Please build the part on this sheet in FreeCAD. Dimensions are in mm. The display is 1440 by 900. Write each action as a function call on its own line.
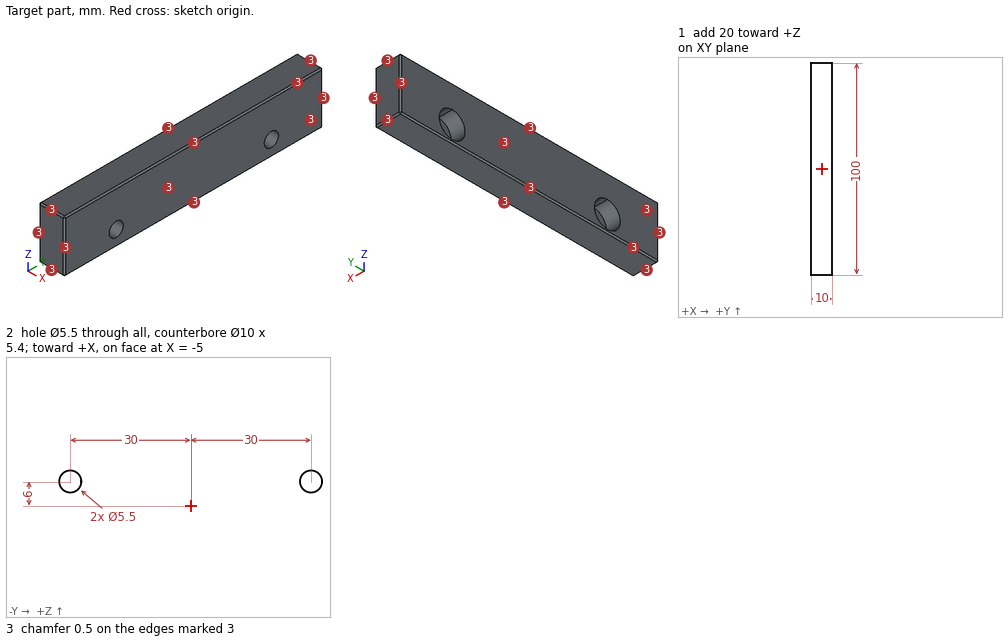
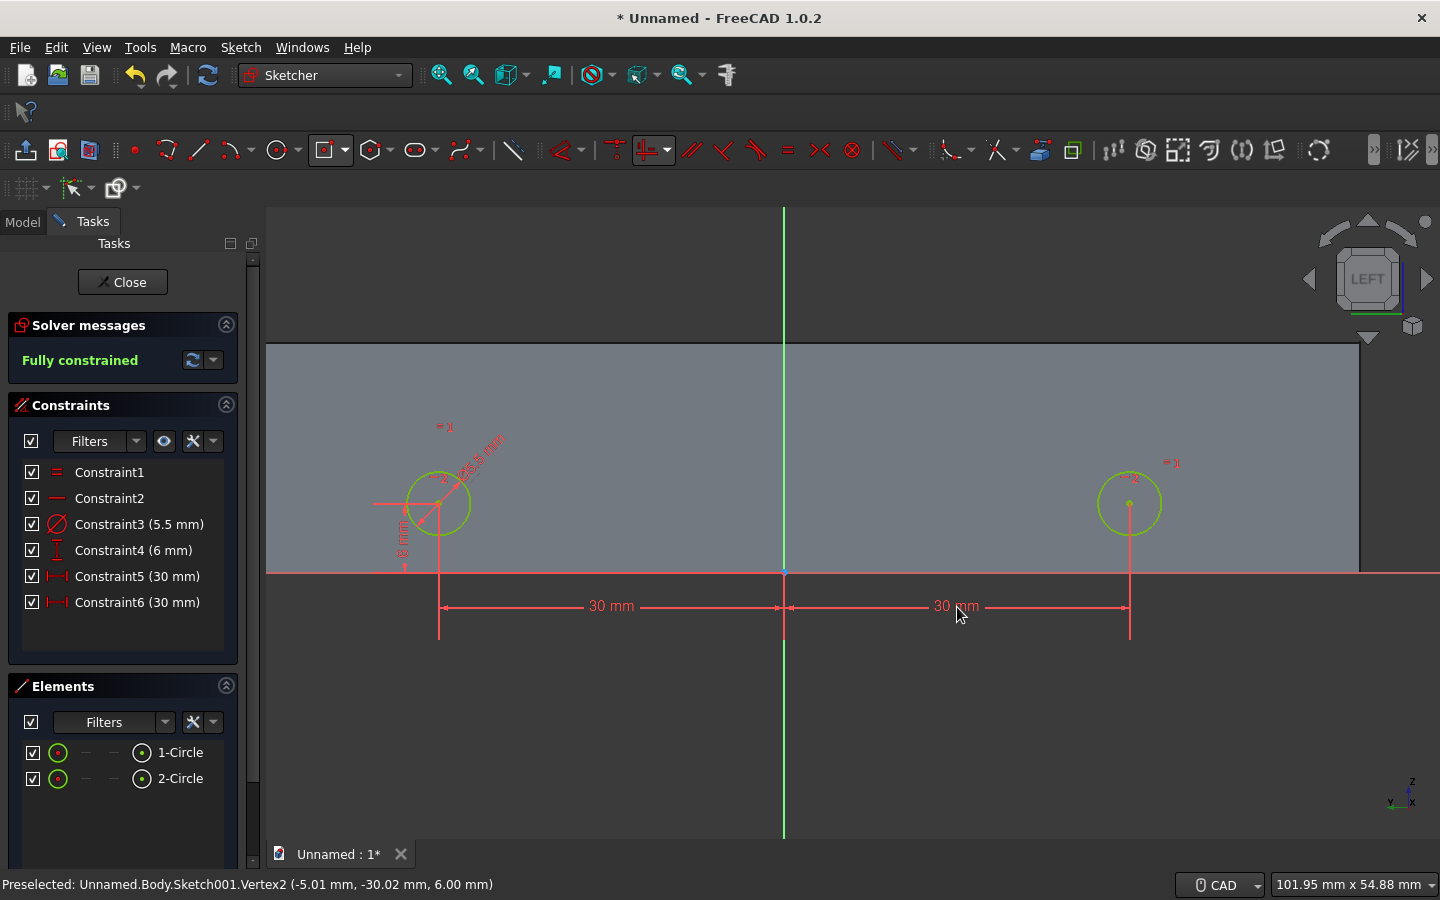
click(123, 282)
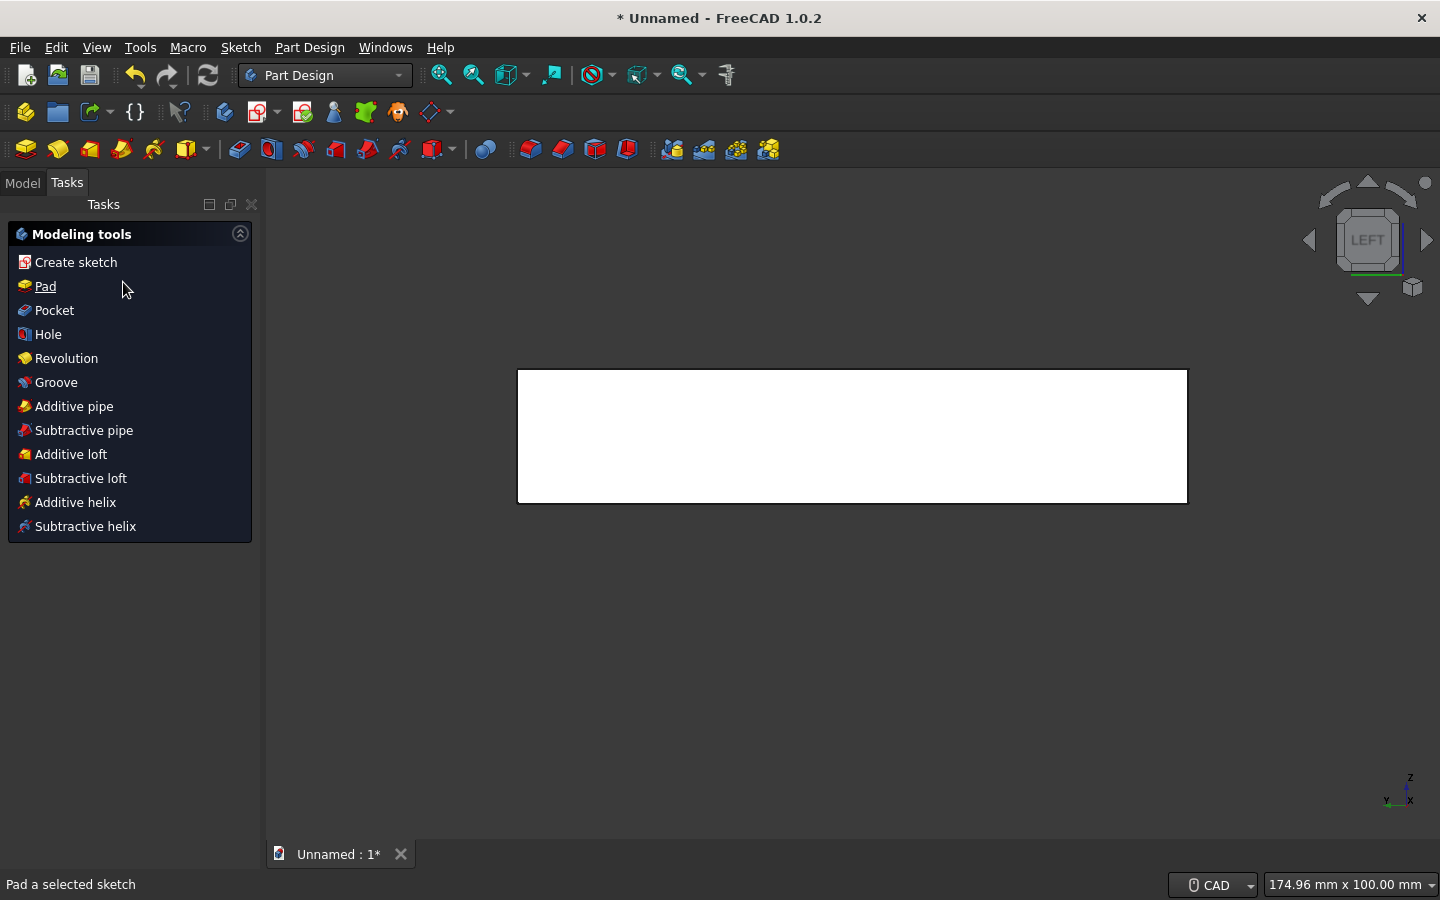
click(272, 150)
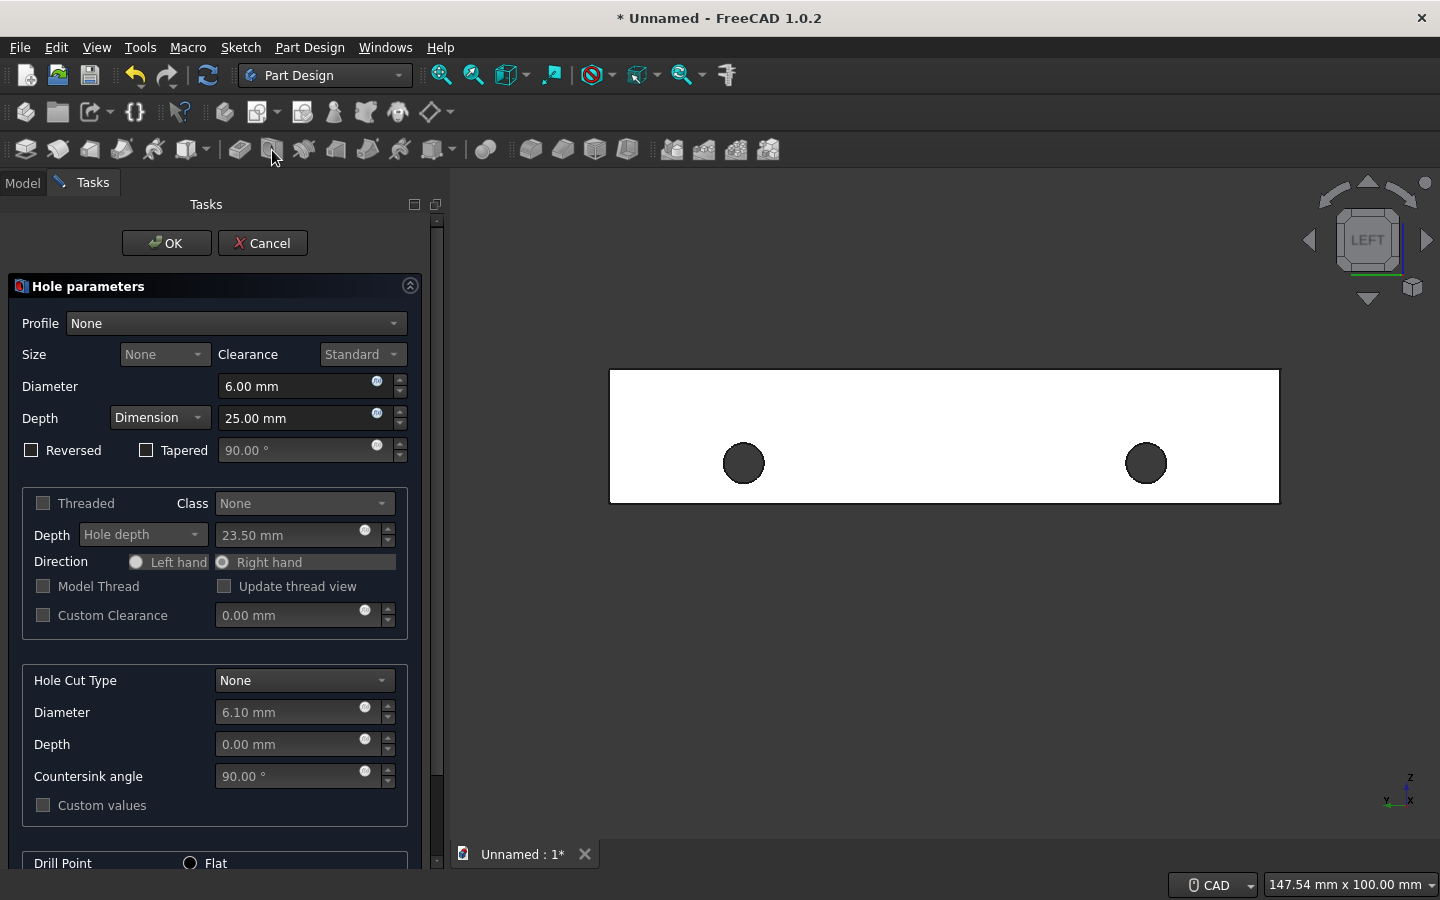
triple_click(305, 386)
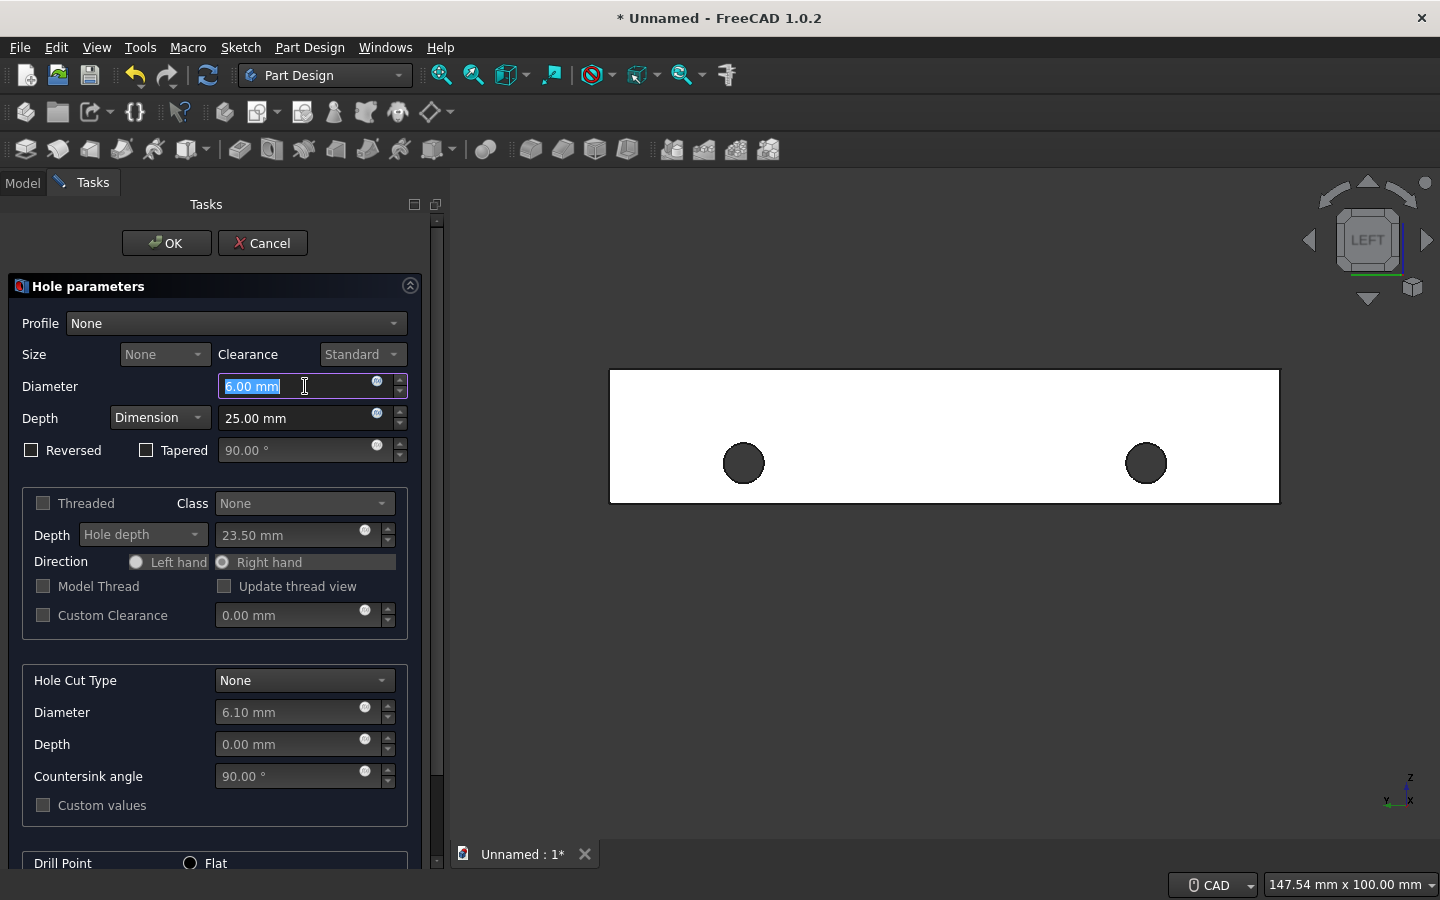
text(5.5)
key(Tab)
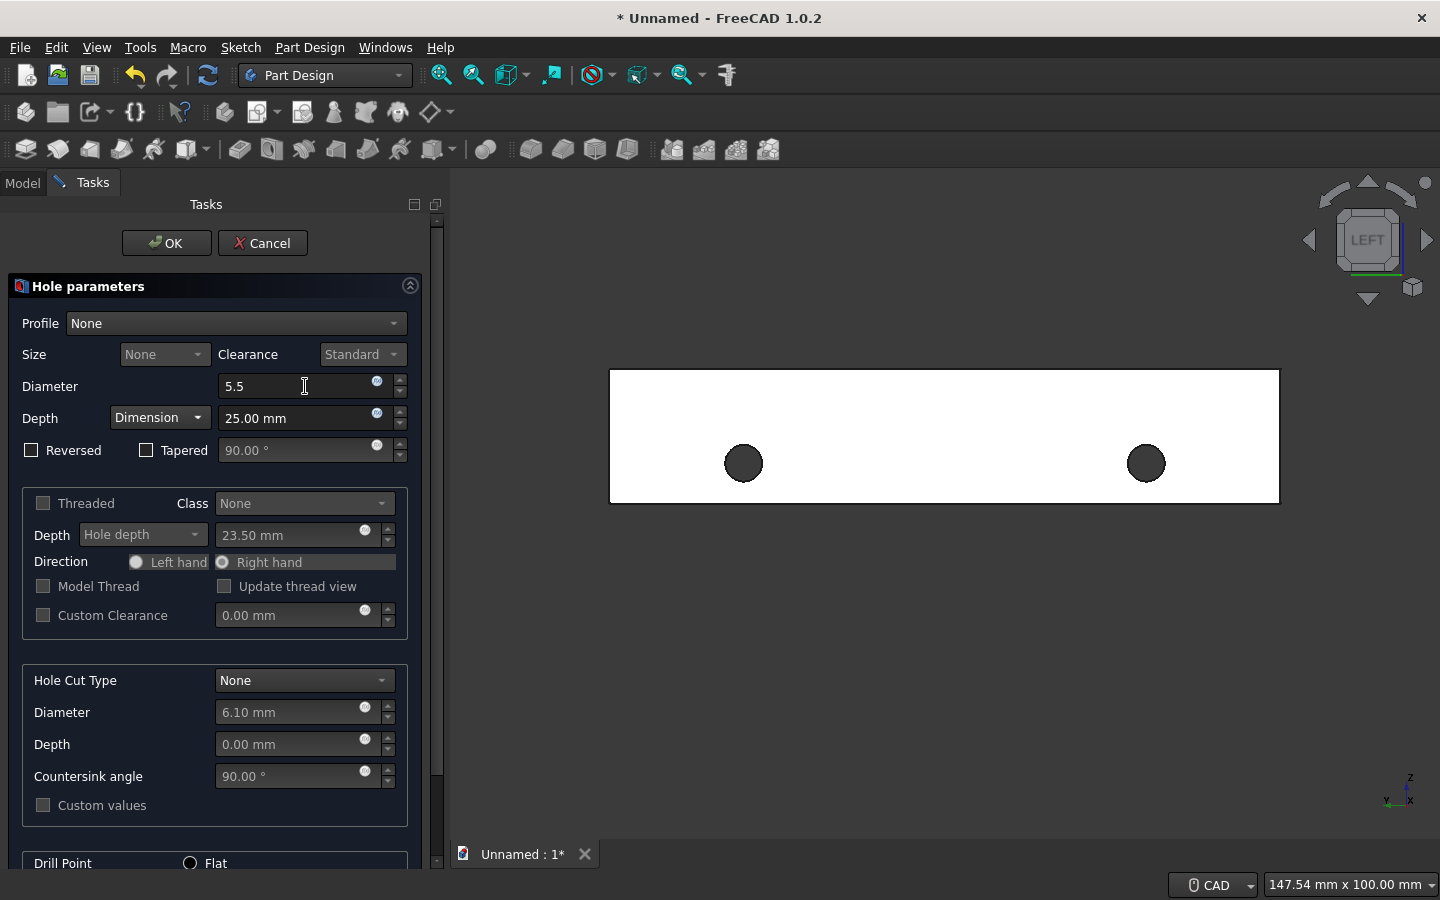
click(161, 418)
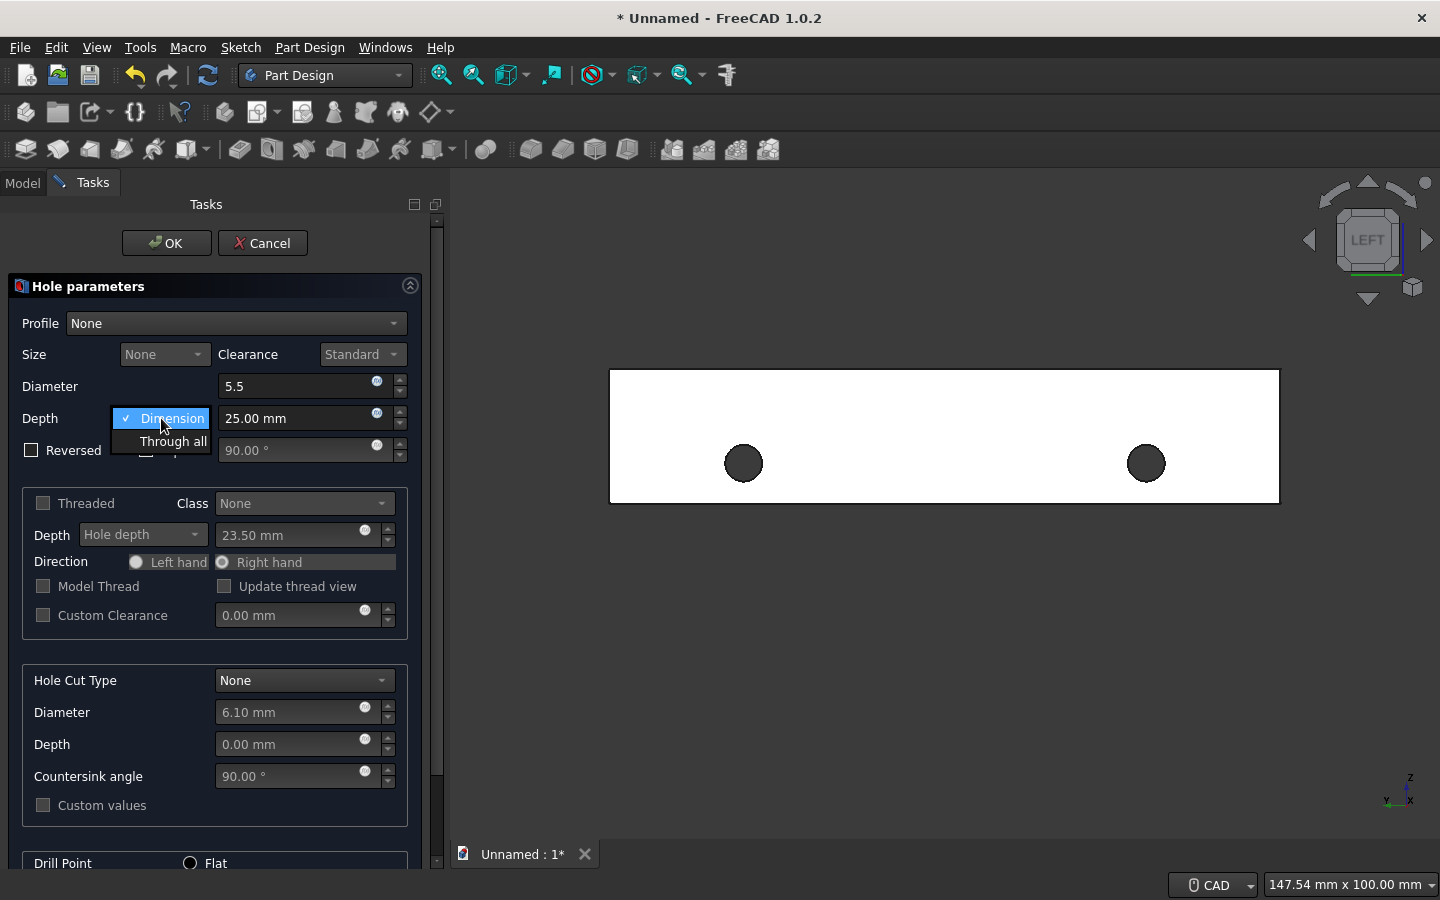
click(160, 442)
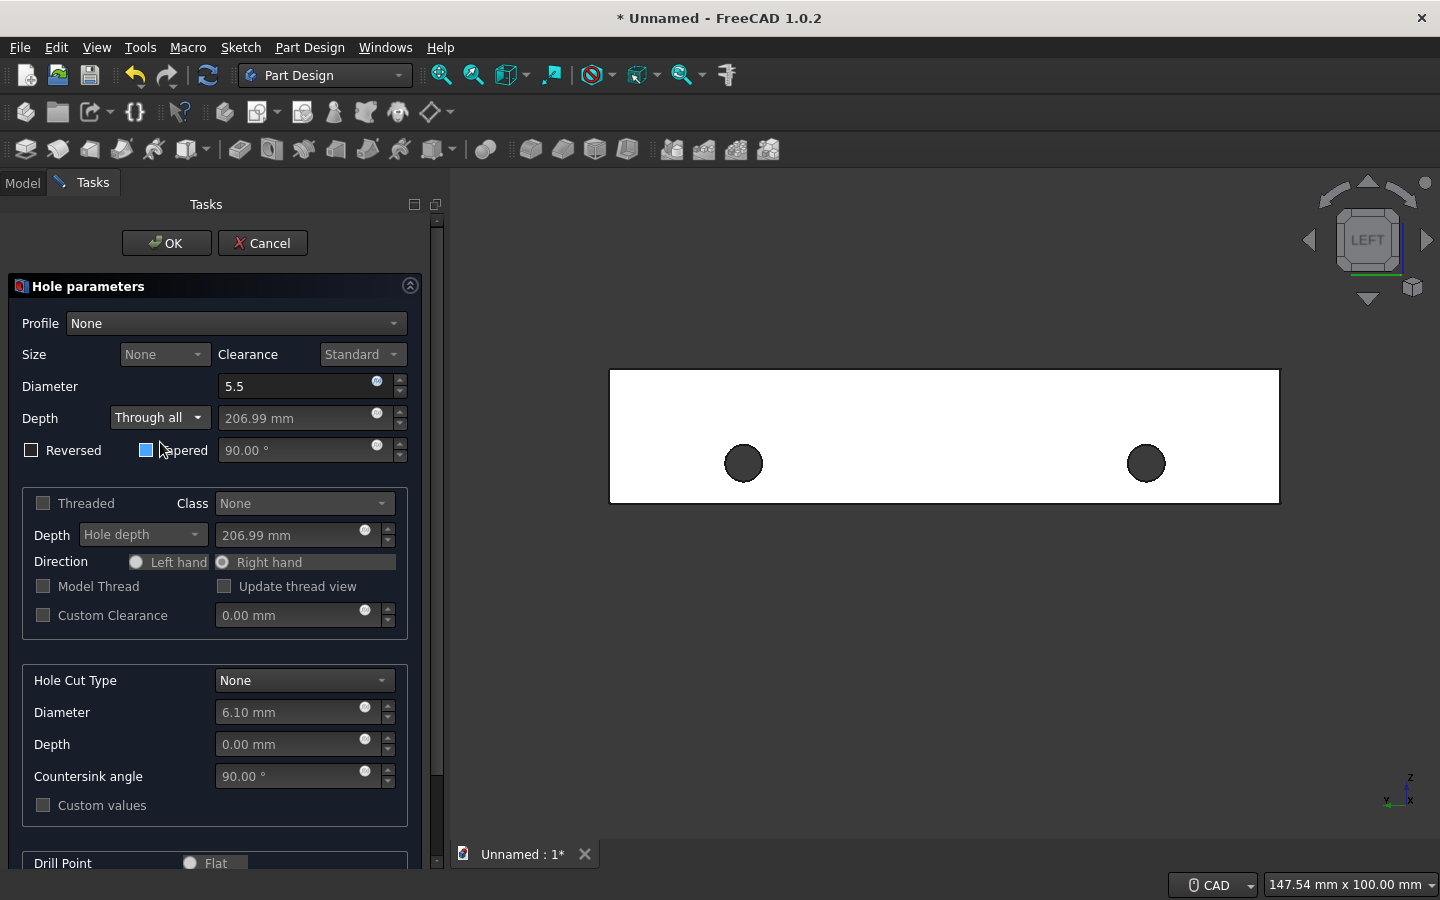
click(306, 680)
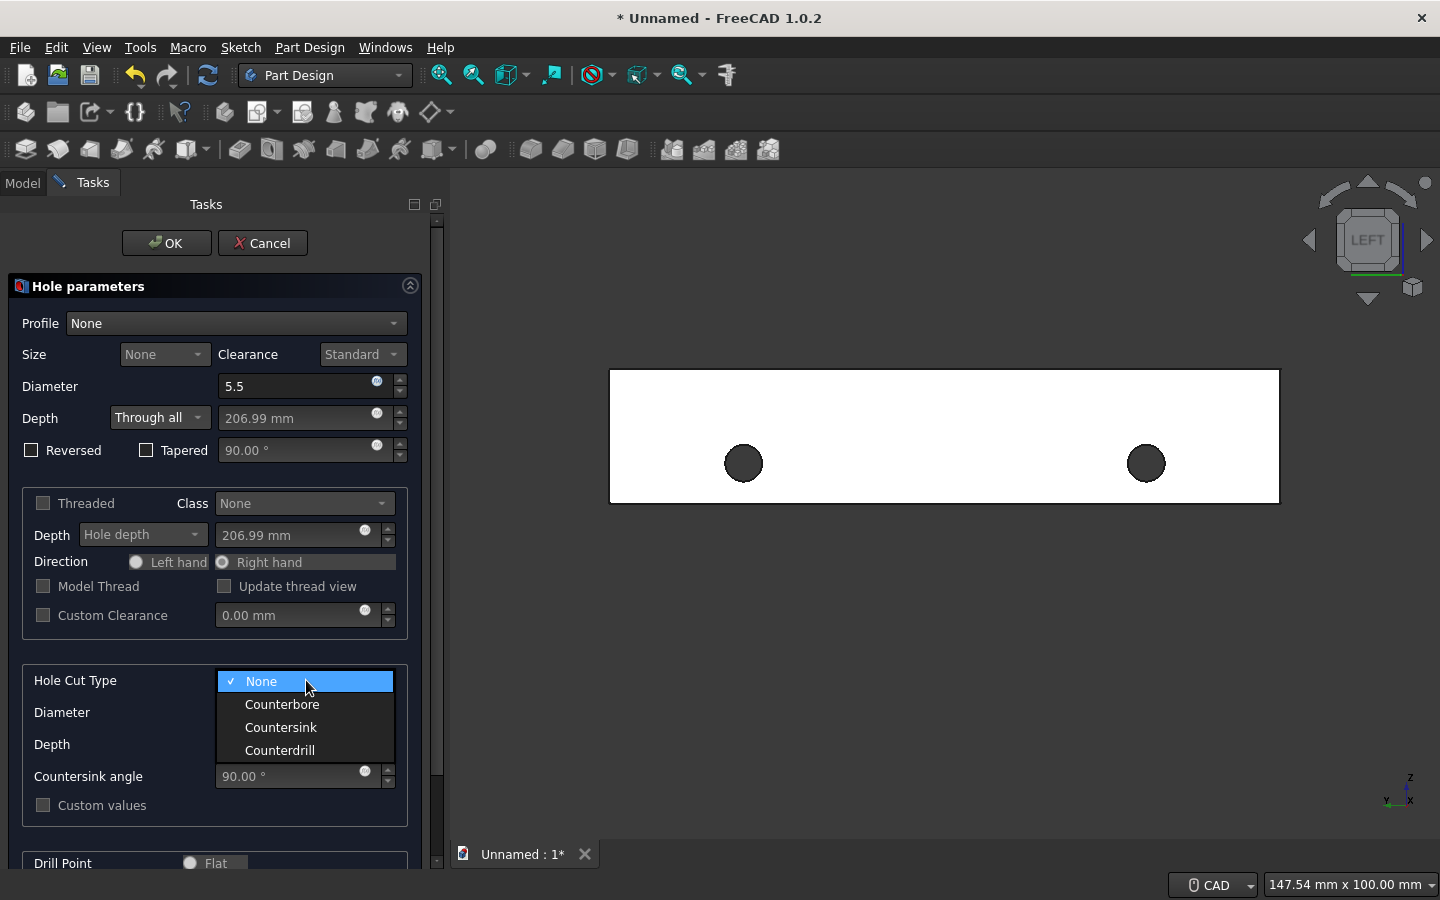
click(304, 704)